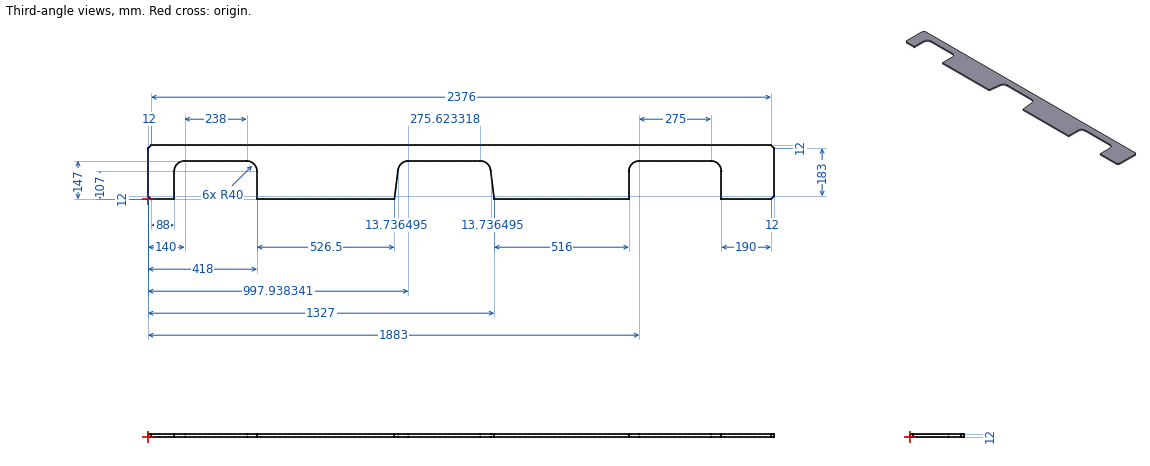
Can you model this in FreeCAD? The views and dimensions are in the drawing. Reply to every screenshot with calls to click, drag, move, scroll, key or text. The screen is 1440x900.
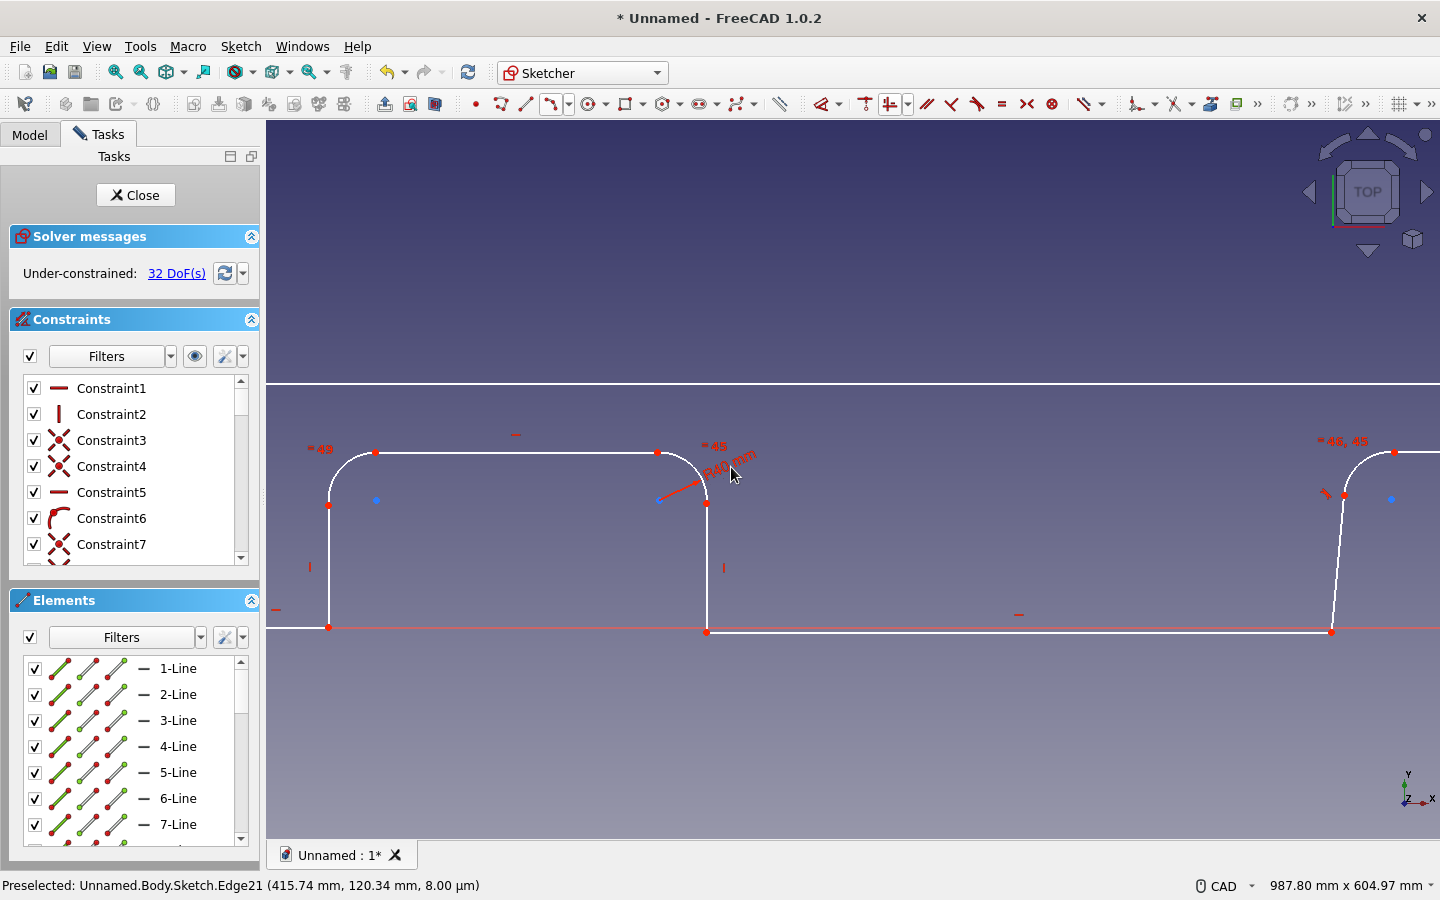
click(707, 633)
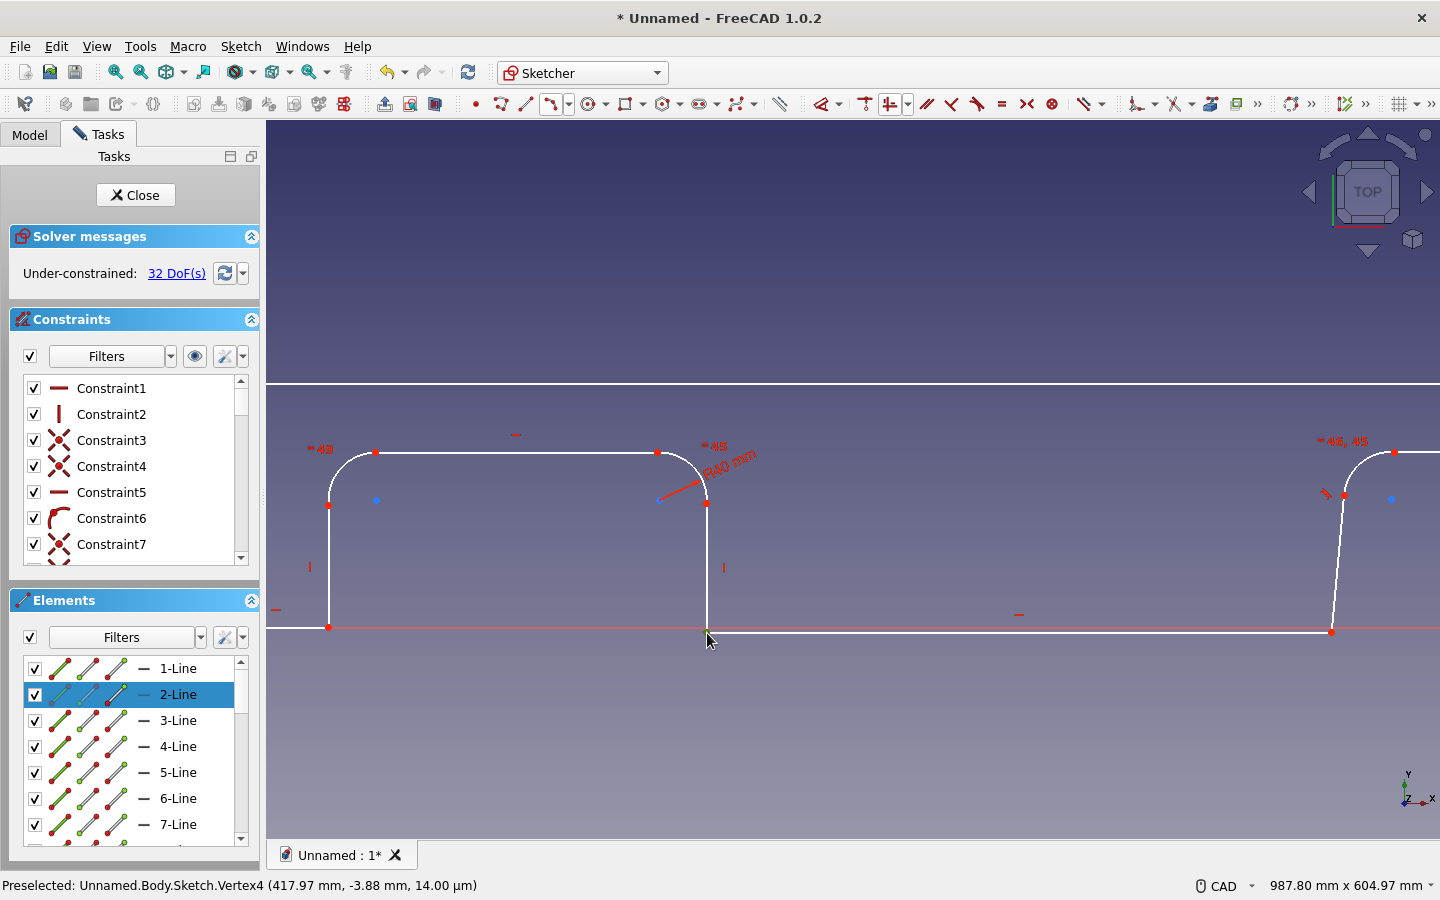
click(364, 628)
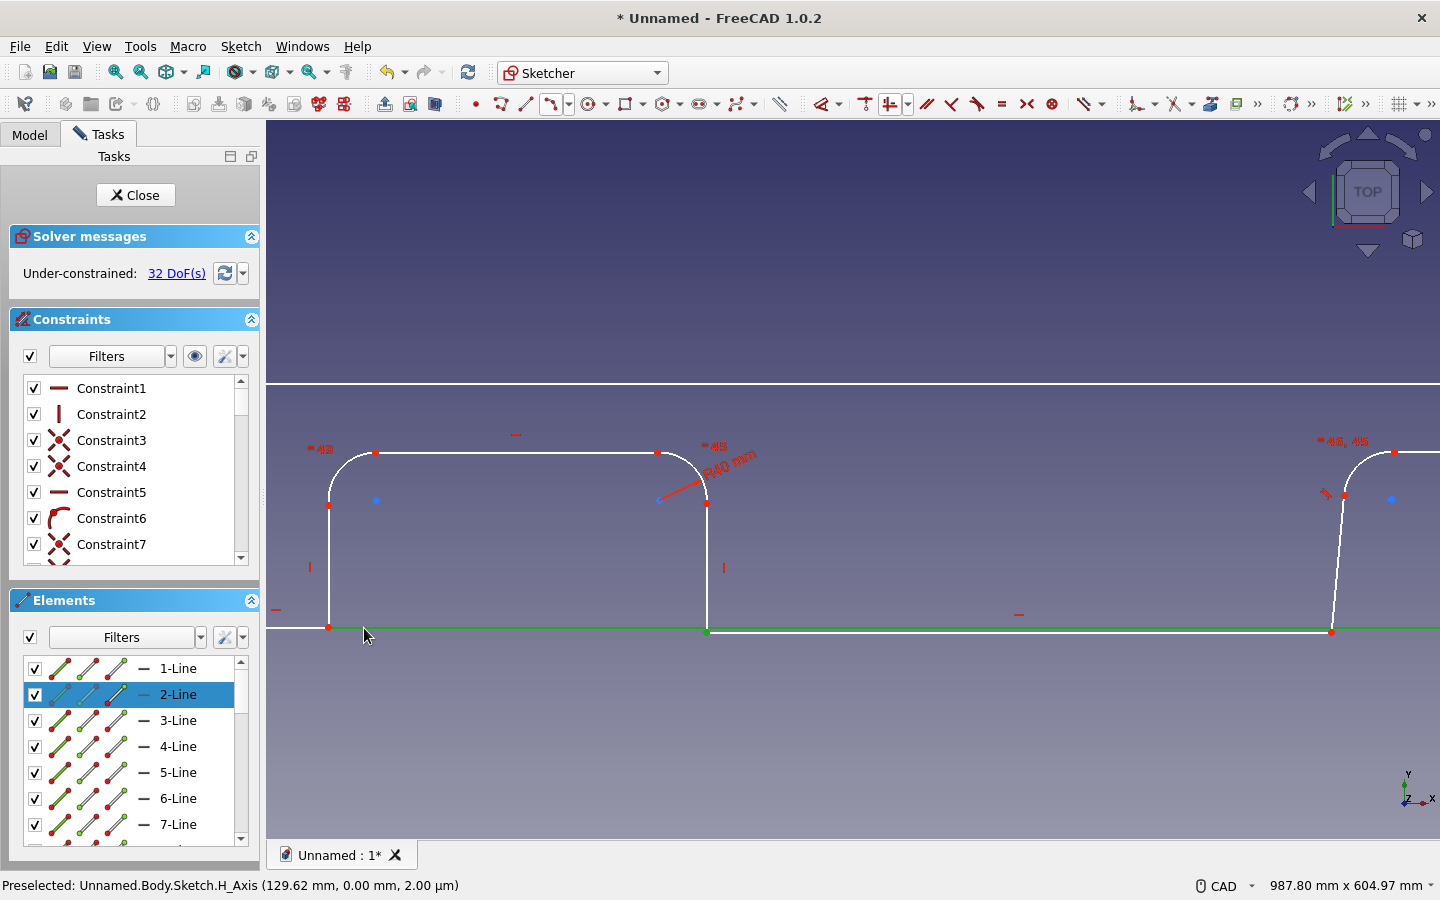
click(865, 104)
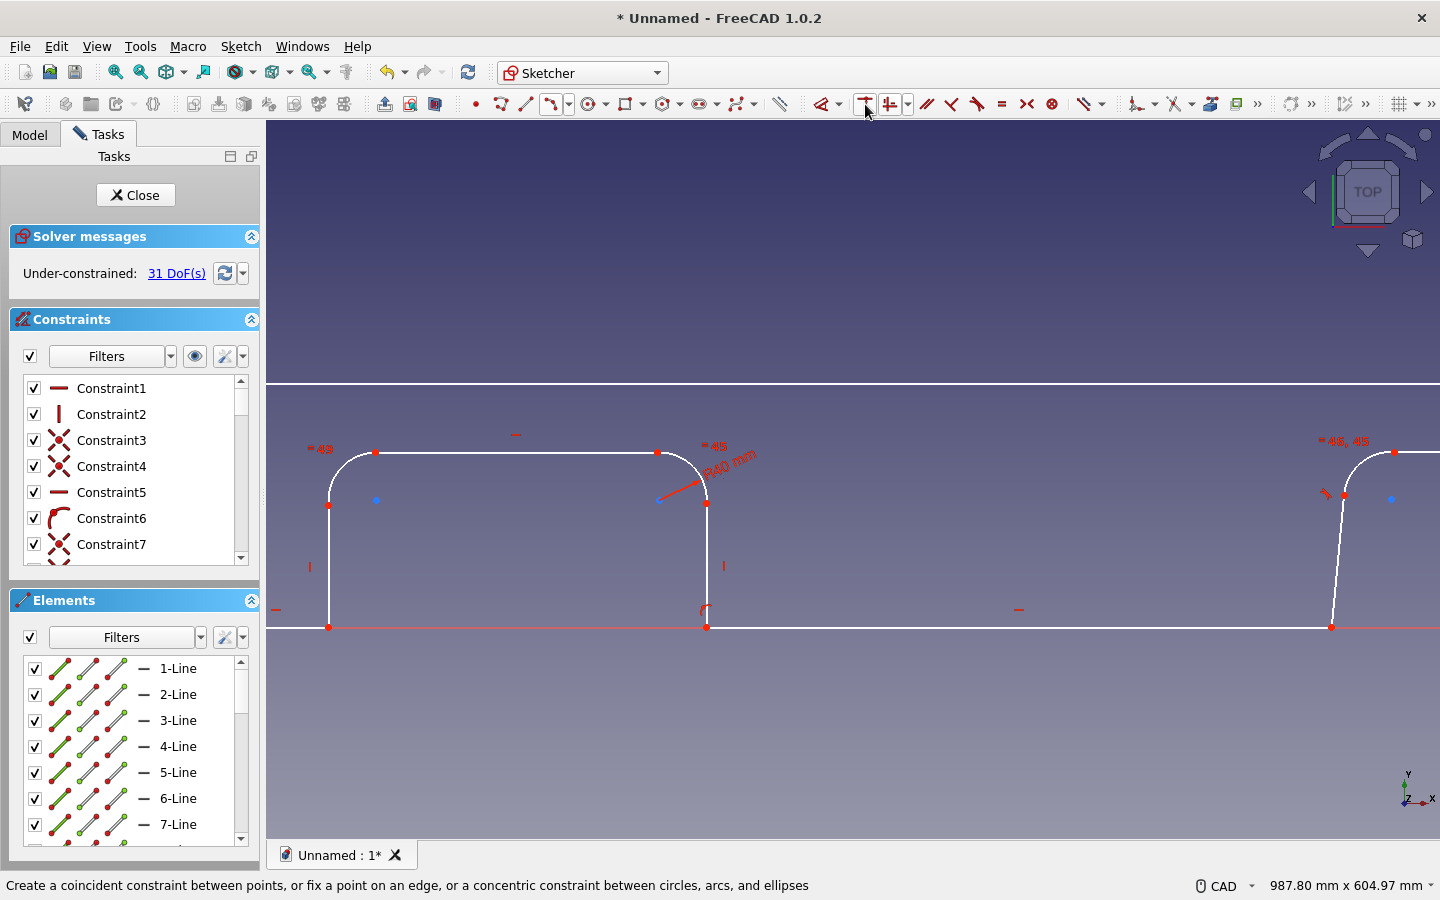
click(820, 104)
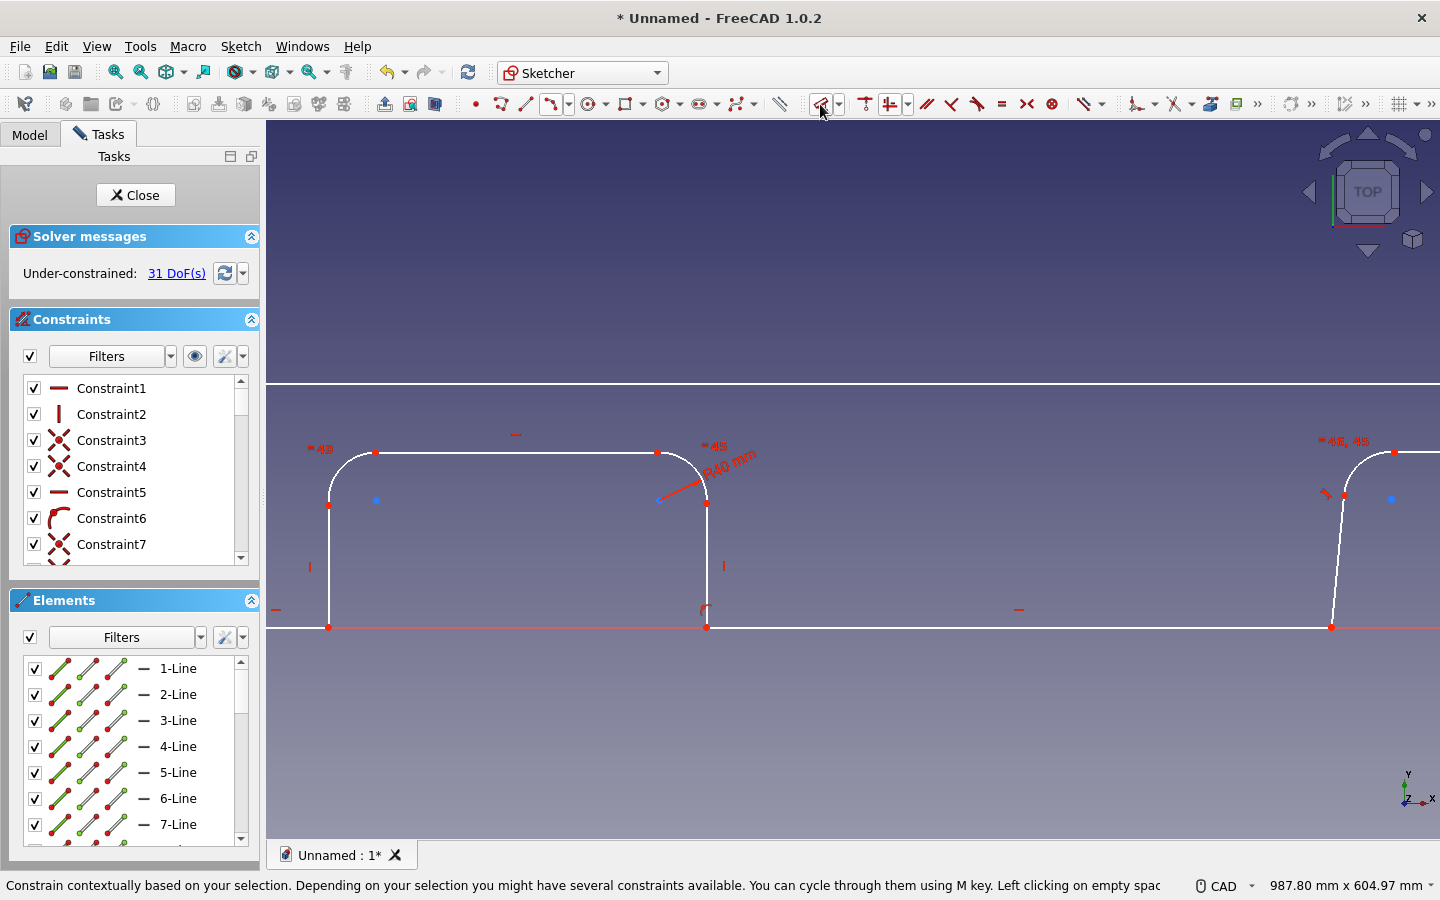
click(297, 628)
click(311, 662)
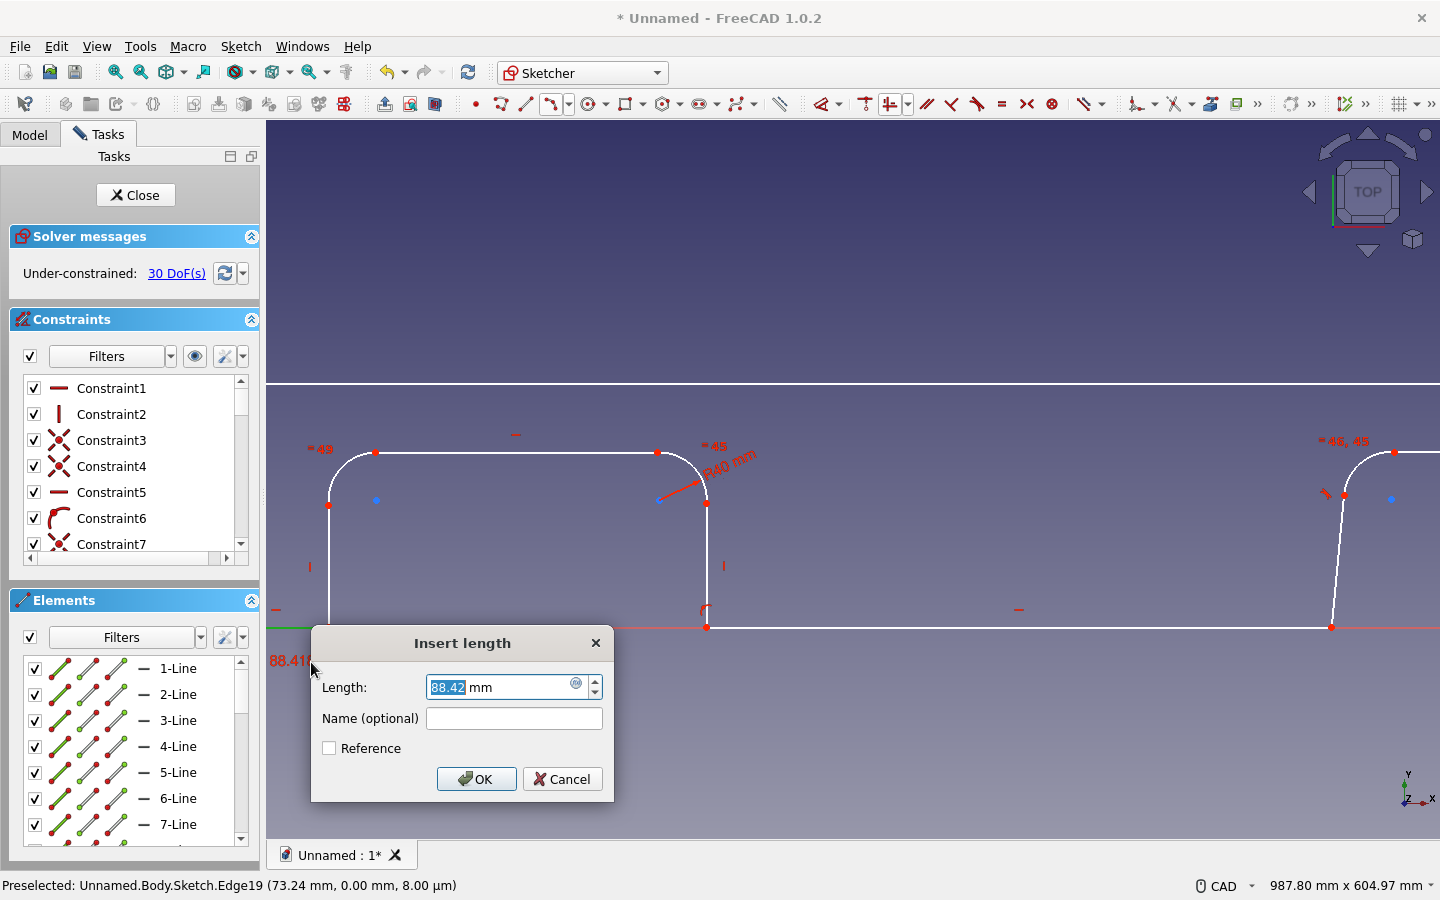
text(88)
key(Return)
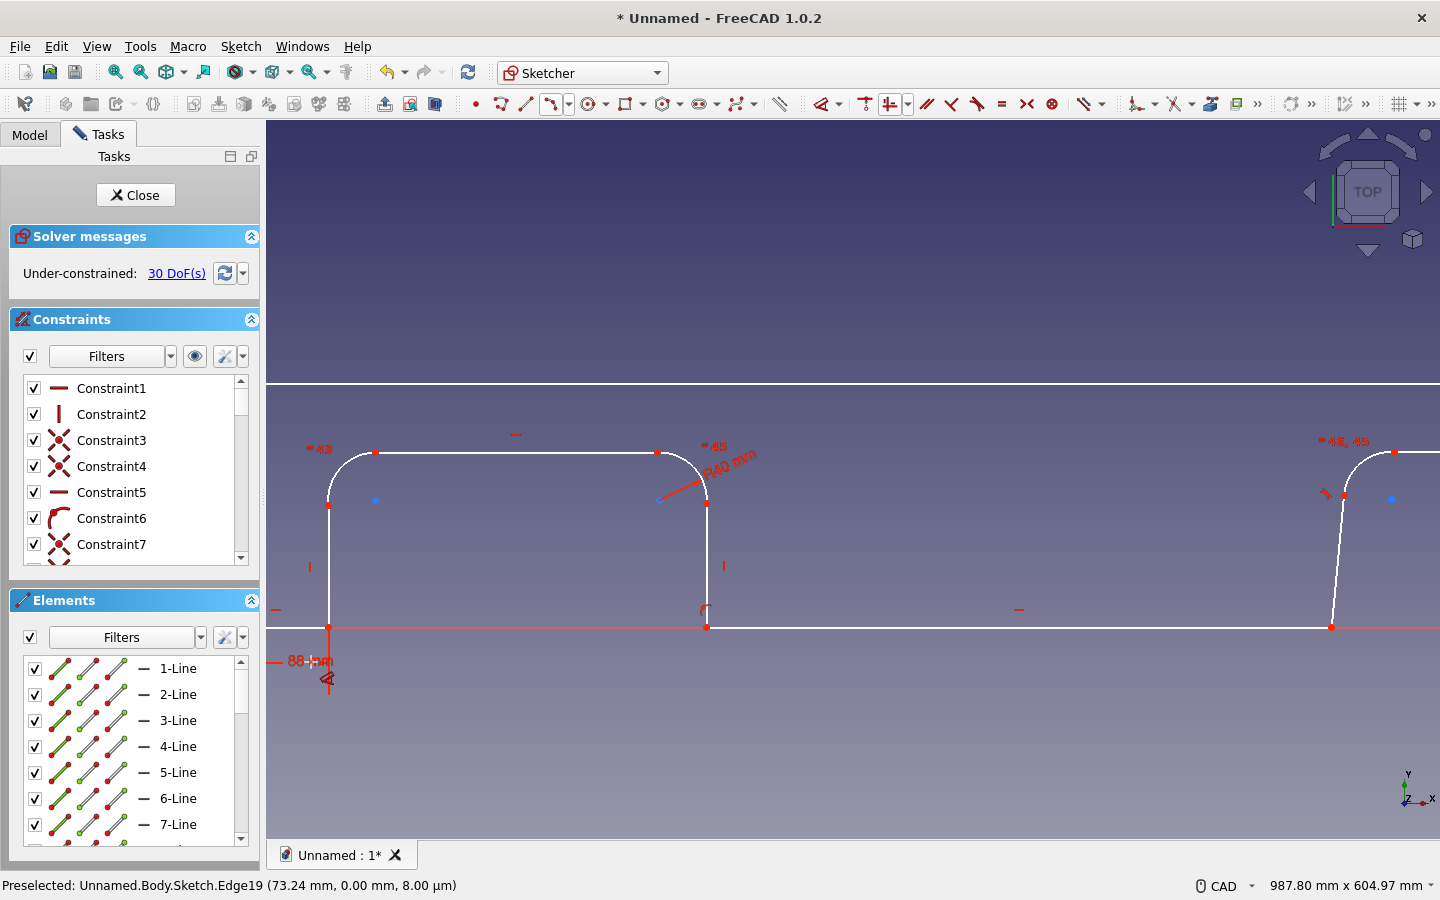
click(460, 453)
click(517, 419)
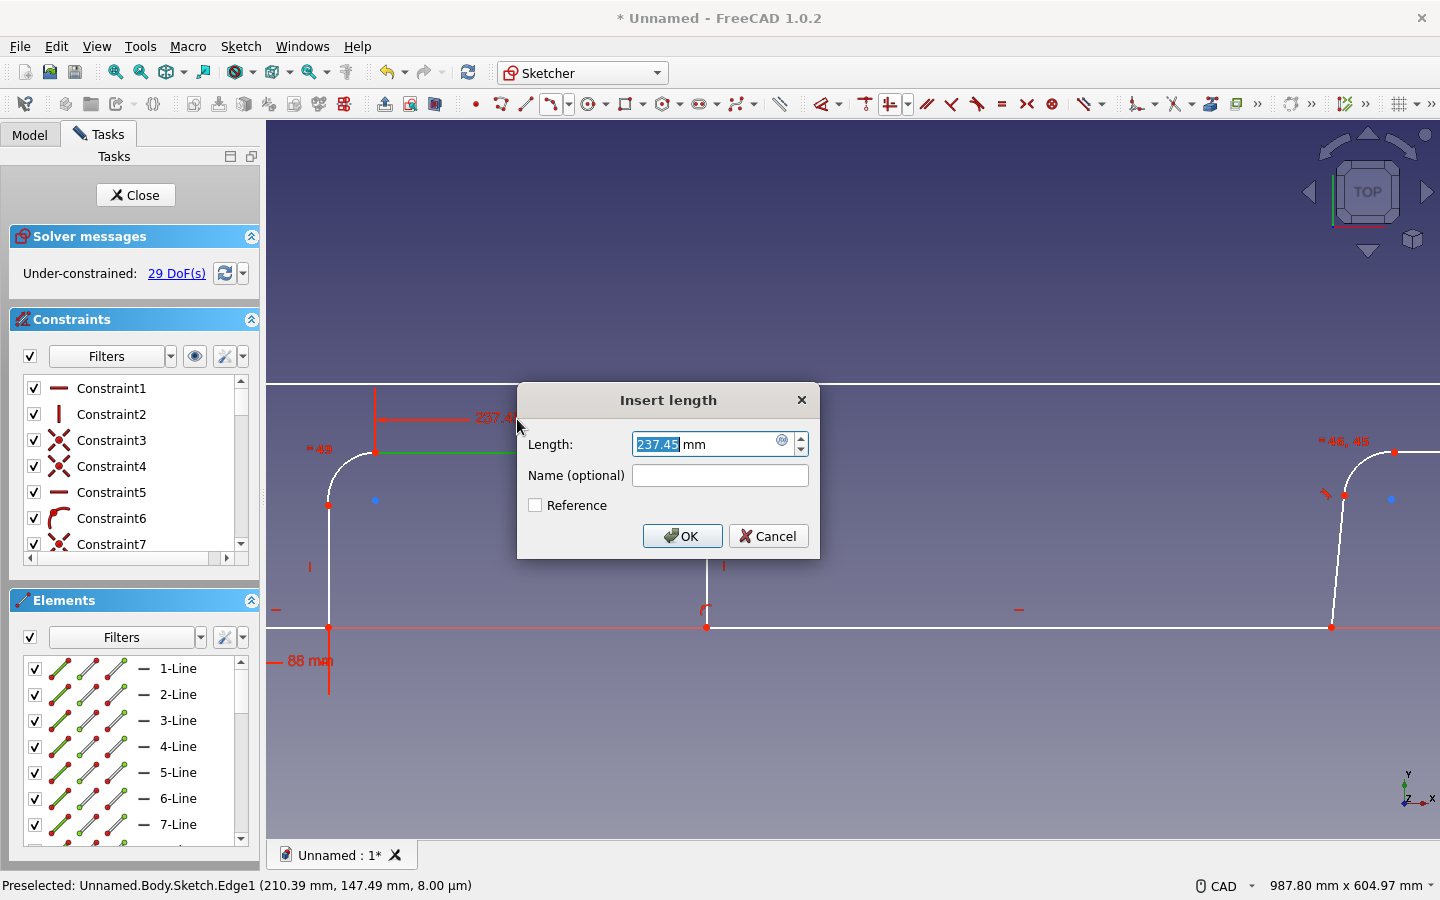
text(238)
key(Return)